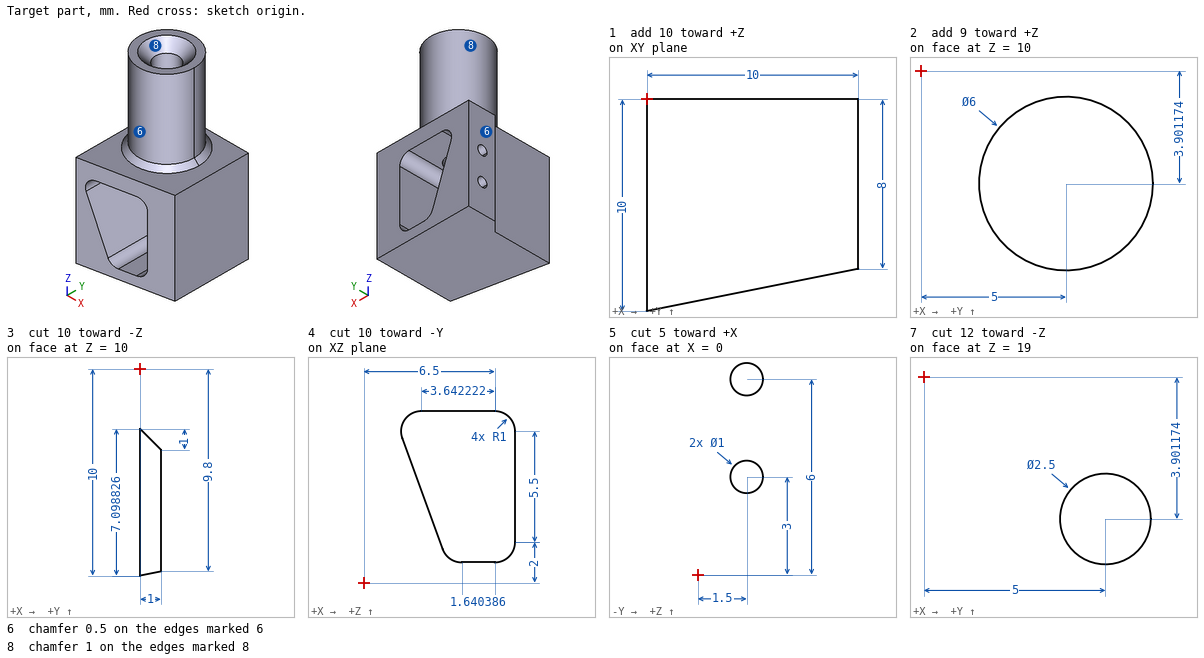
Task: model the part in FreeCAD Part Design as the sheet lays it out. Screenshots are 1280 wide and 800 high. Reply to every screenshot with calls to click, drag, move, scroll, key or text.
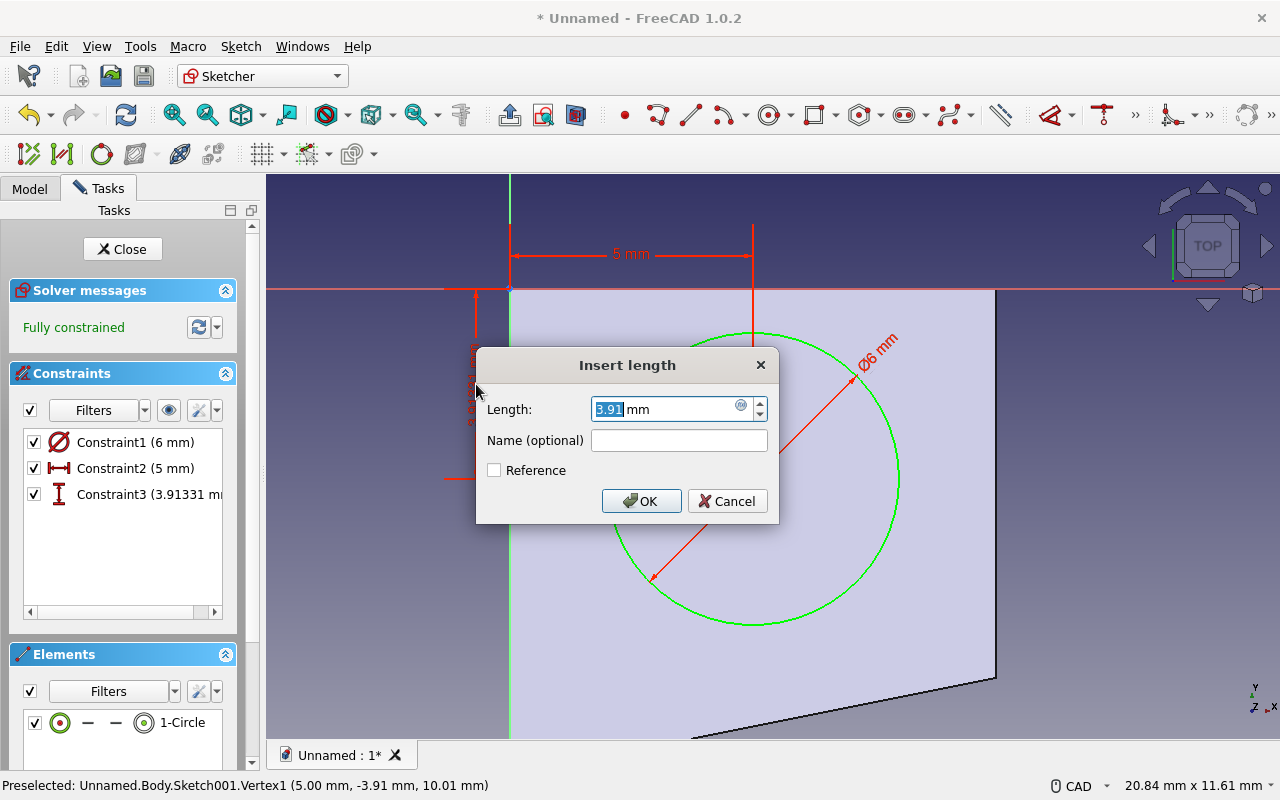
text(3.901174)
key(Return)
key(Escape)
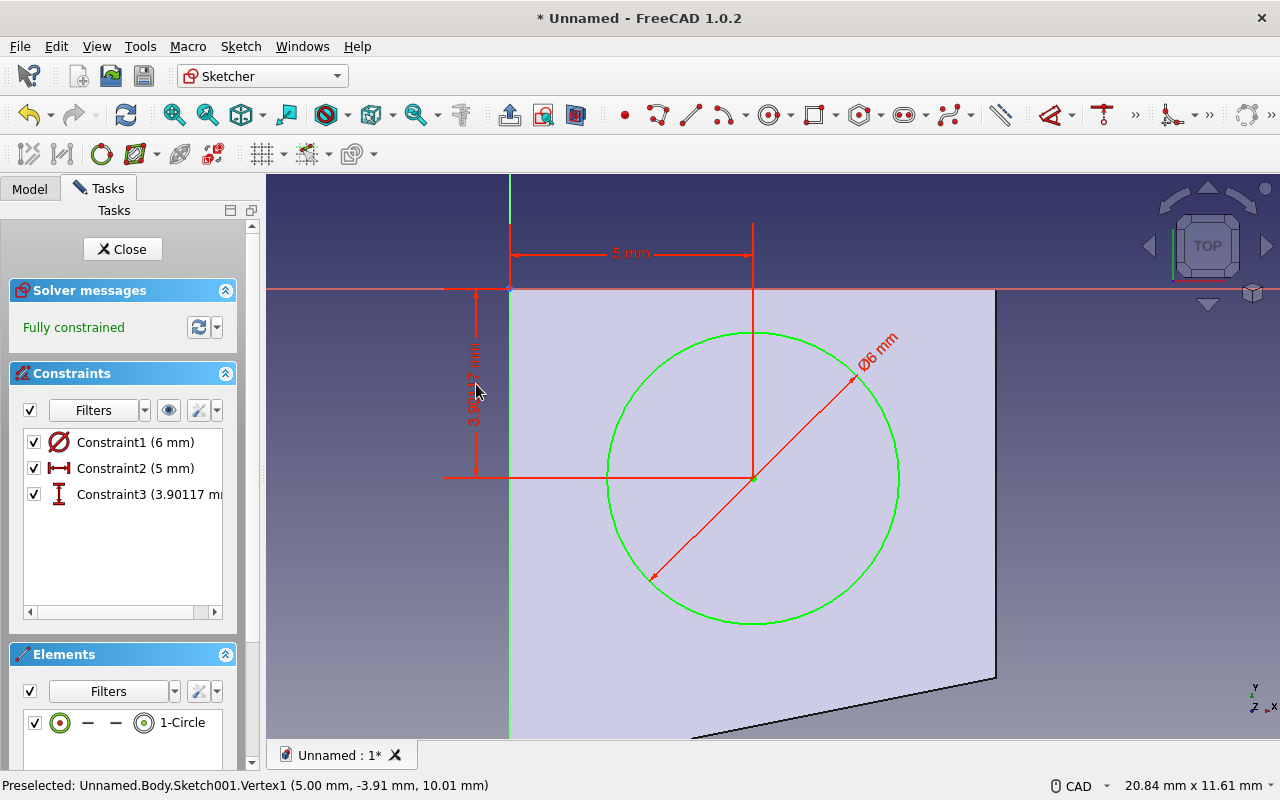
click(123, 249)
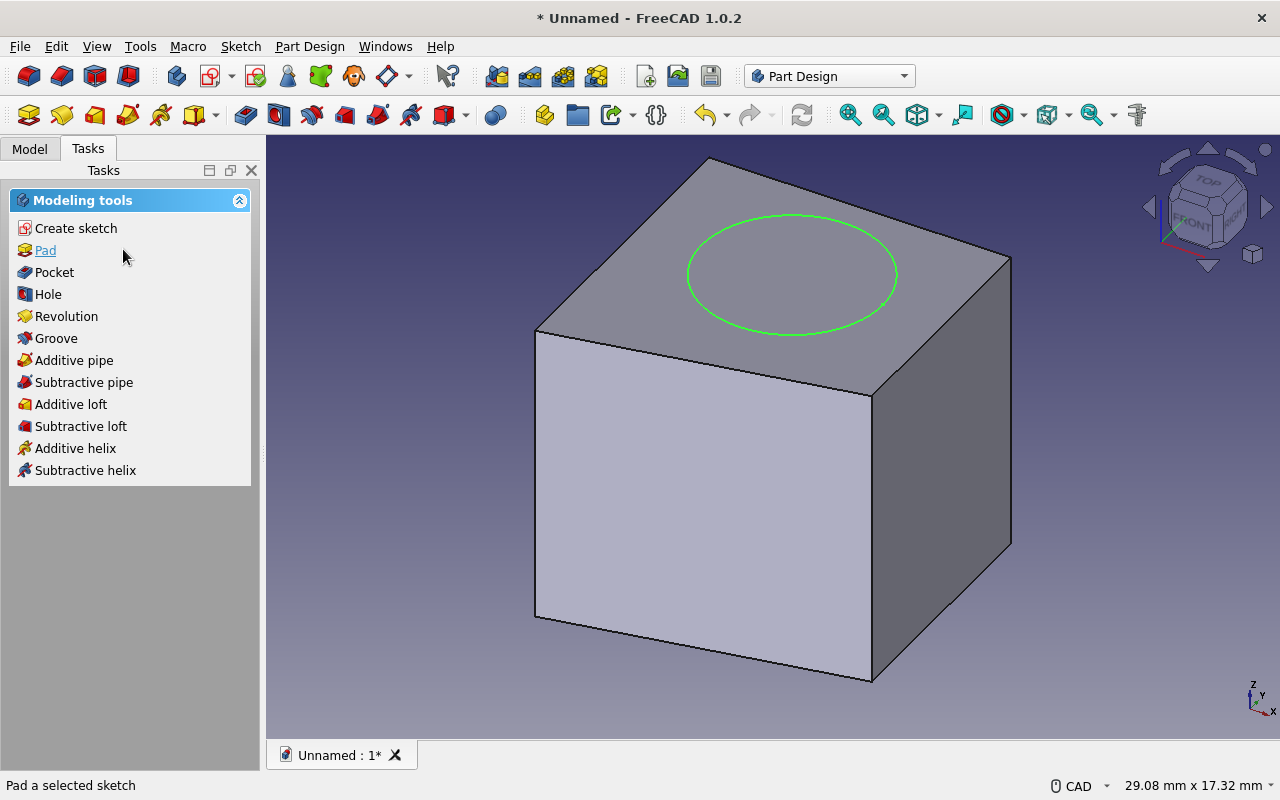
click(29, 116)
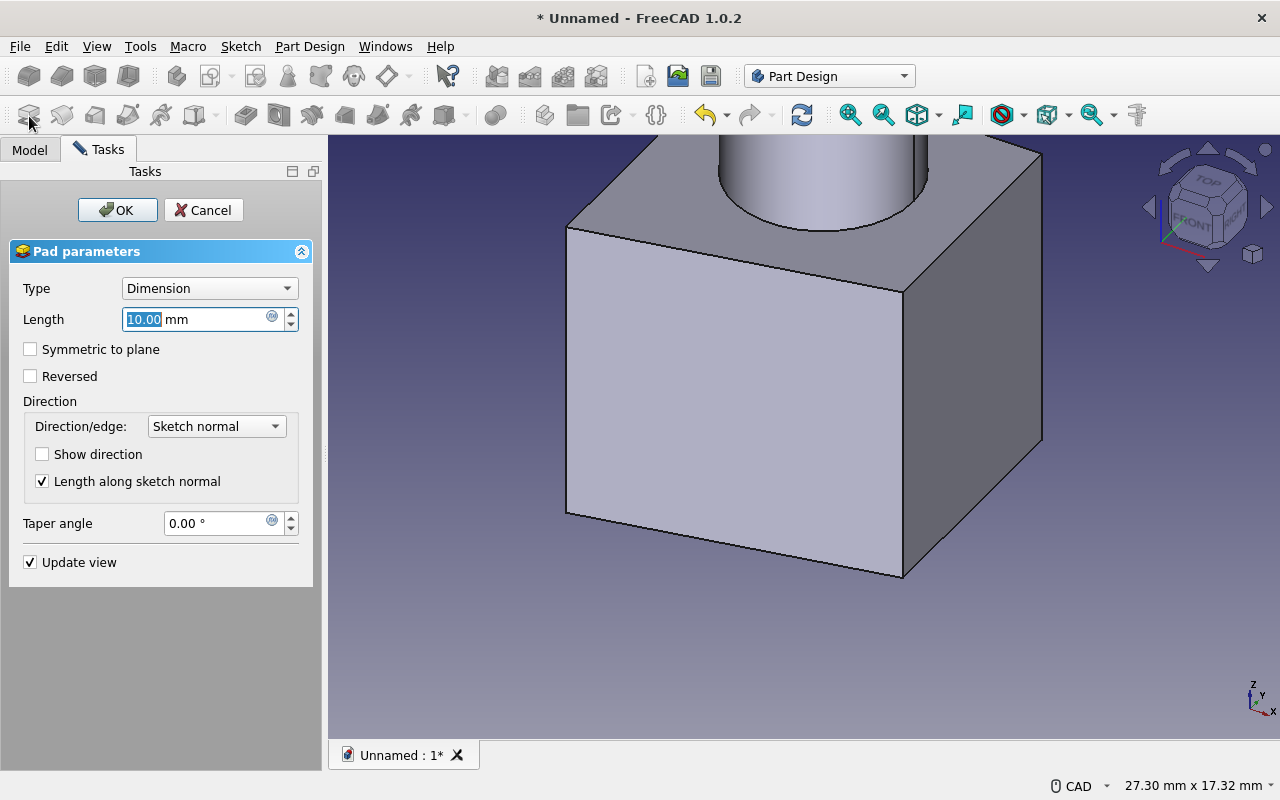
text(9)
key(Tab)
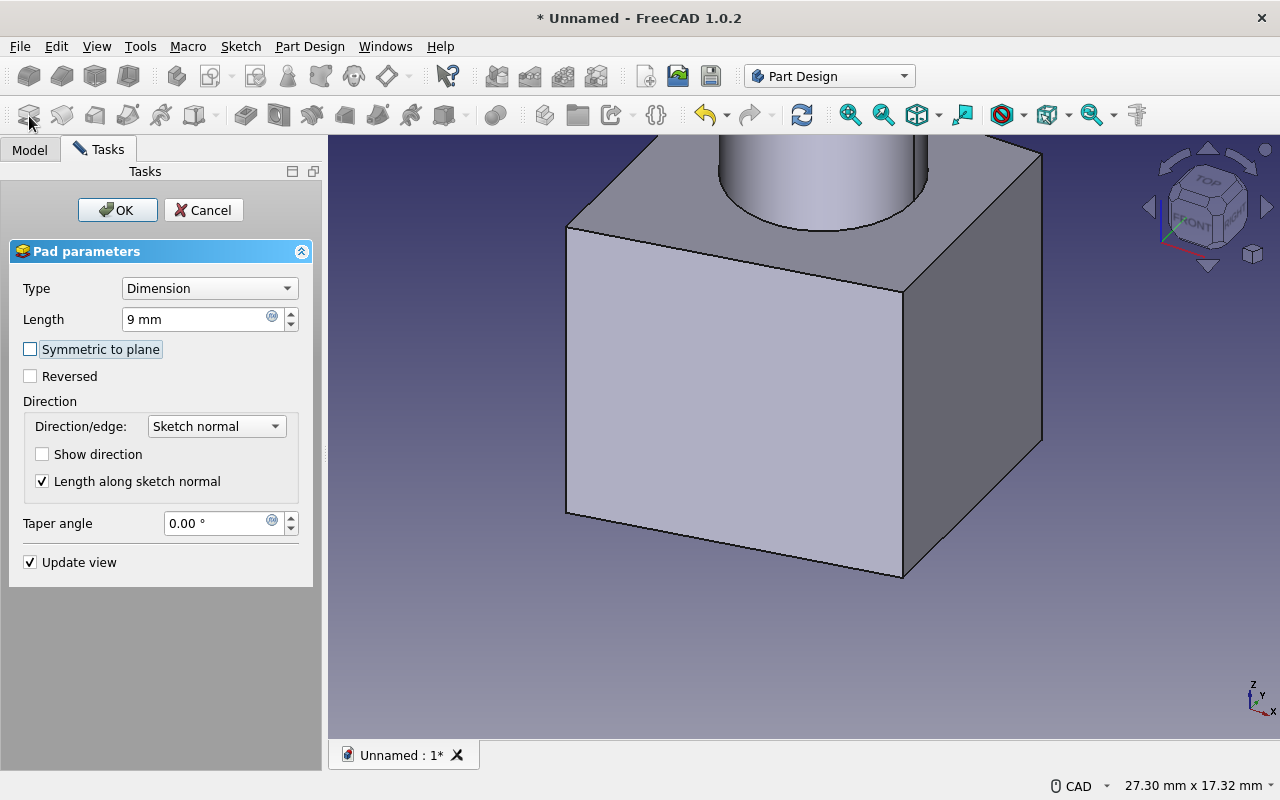
click(118, 210)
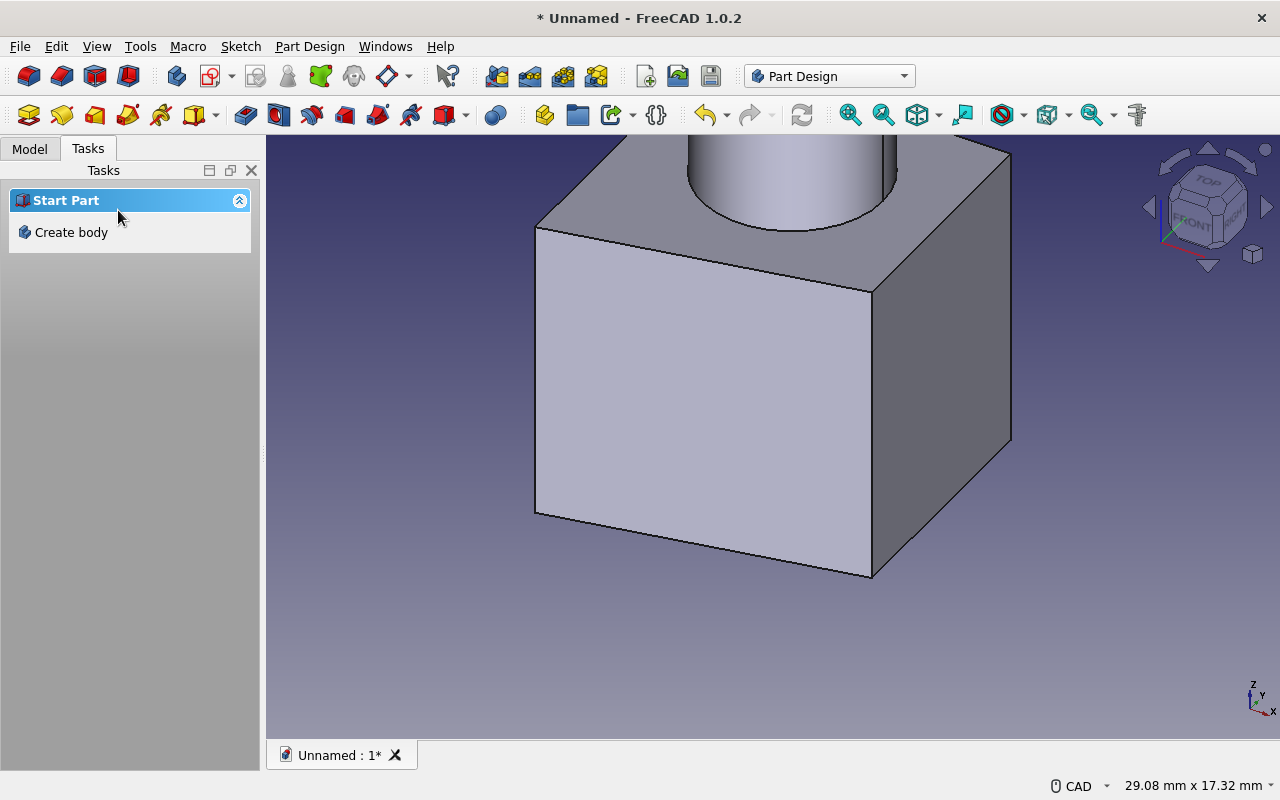
key(v)
key(f)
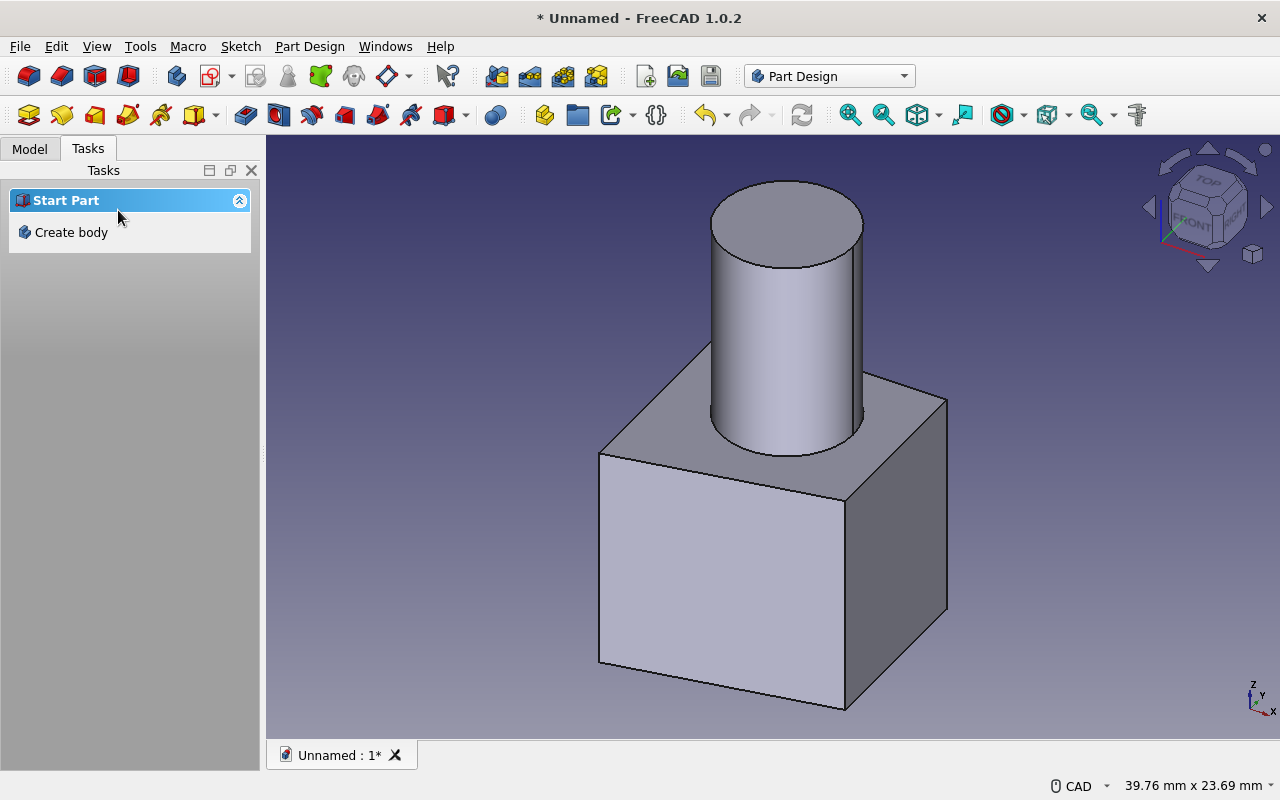
click(673, 441)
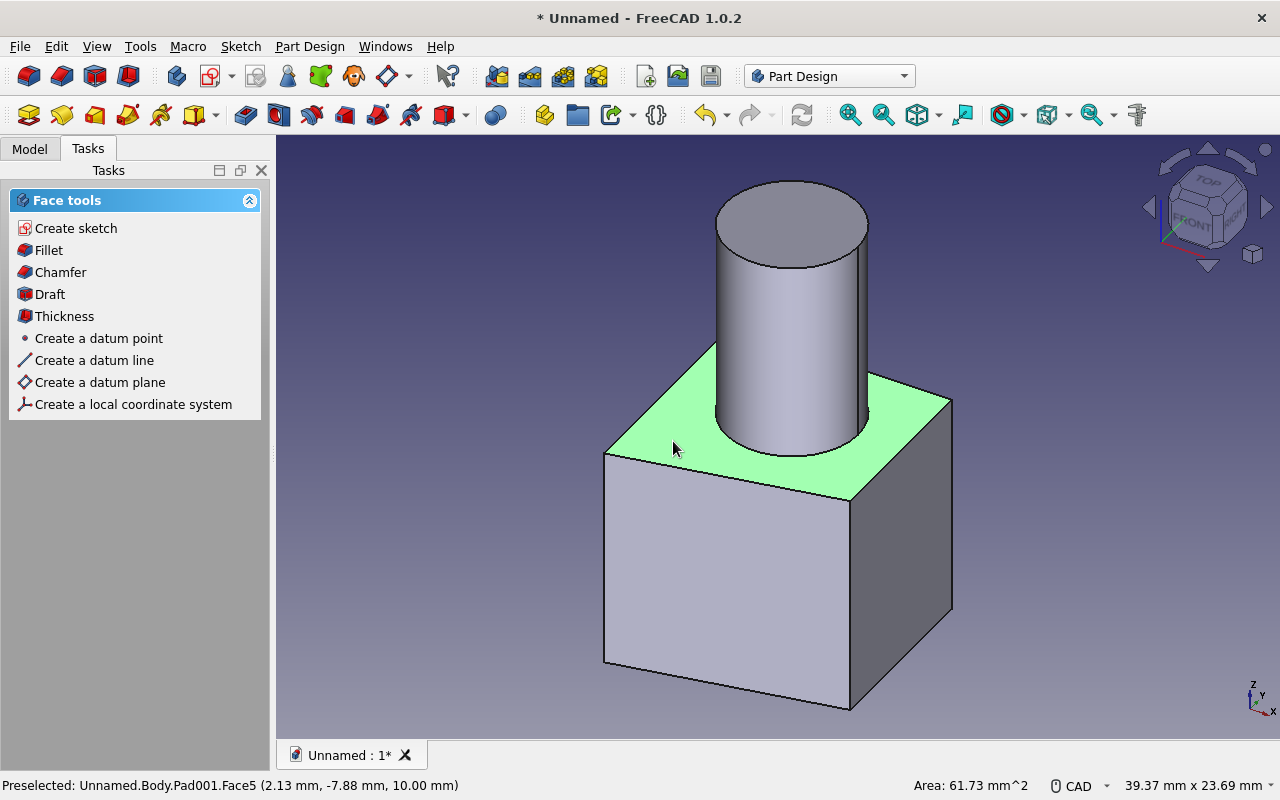
click(210, 76)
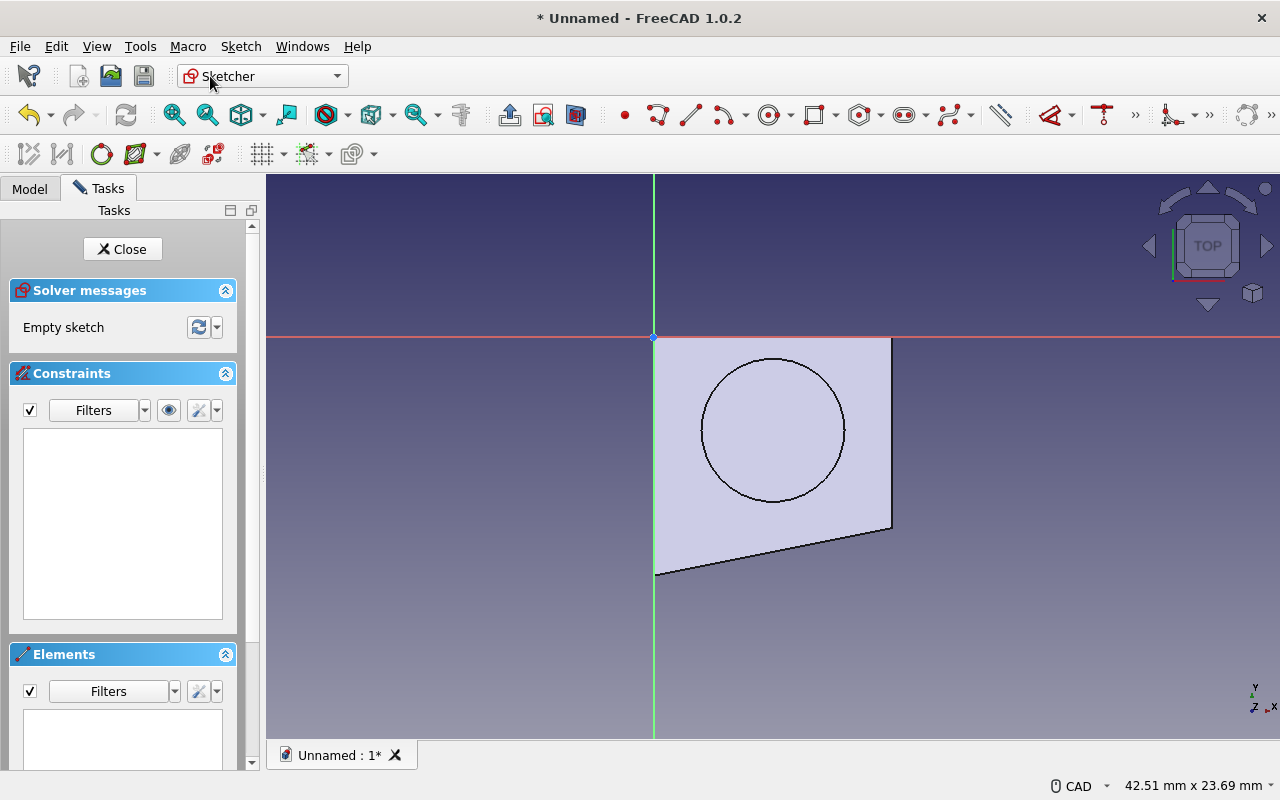
scroll(587, 456, up, 2)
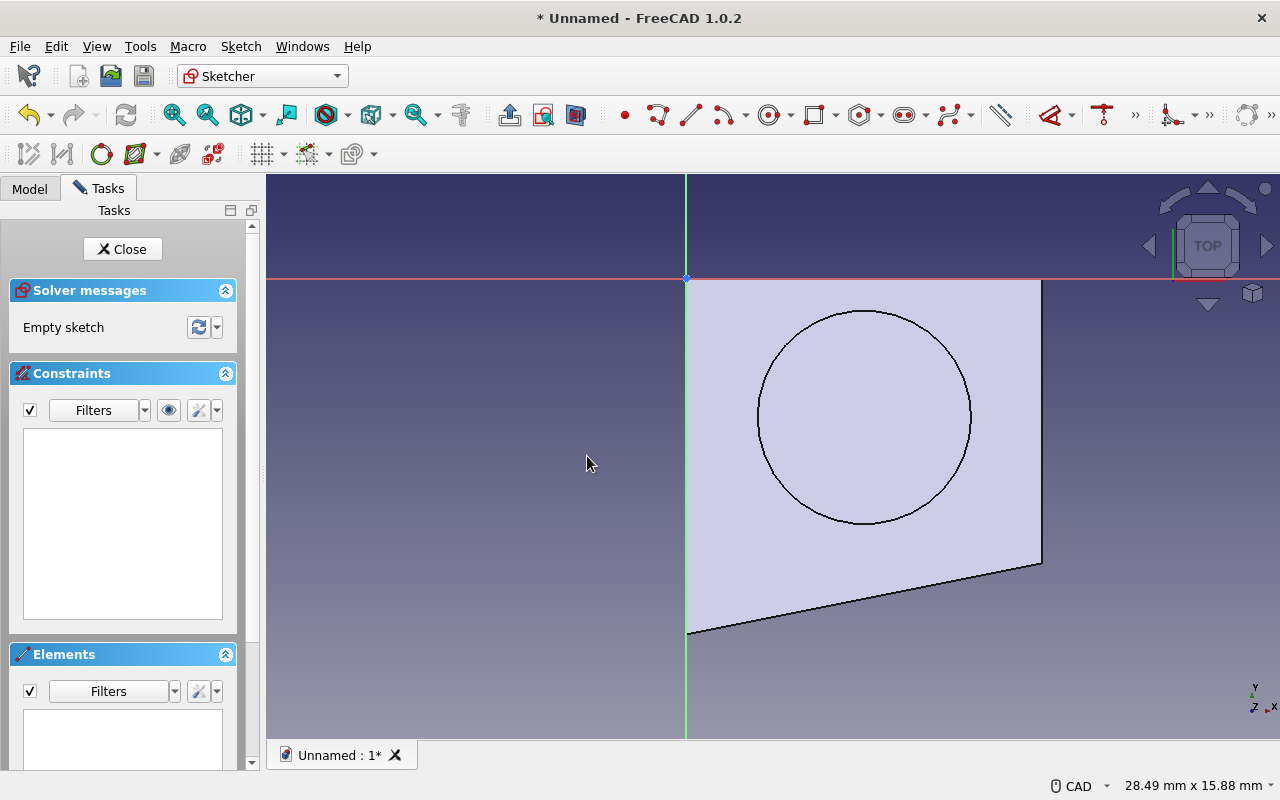
key(g)
key(m)